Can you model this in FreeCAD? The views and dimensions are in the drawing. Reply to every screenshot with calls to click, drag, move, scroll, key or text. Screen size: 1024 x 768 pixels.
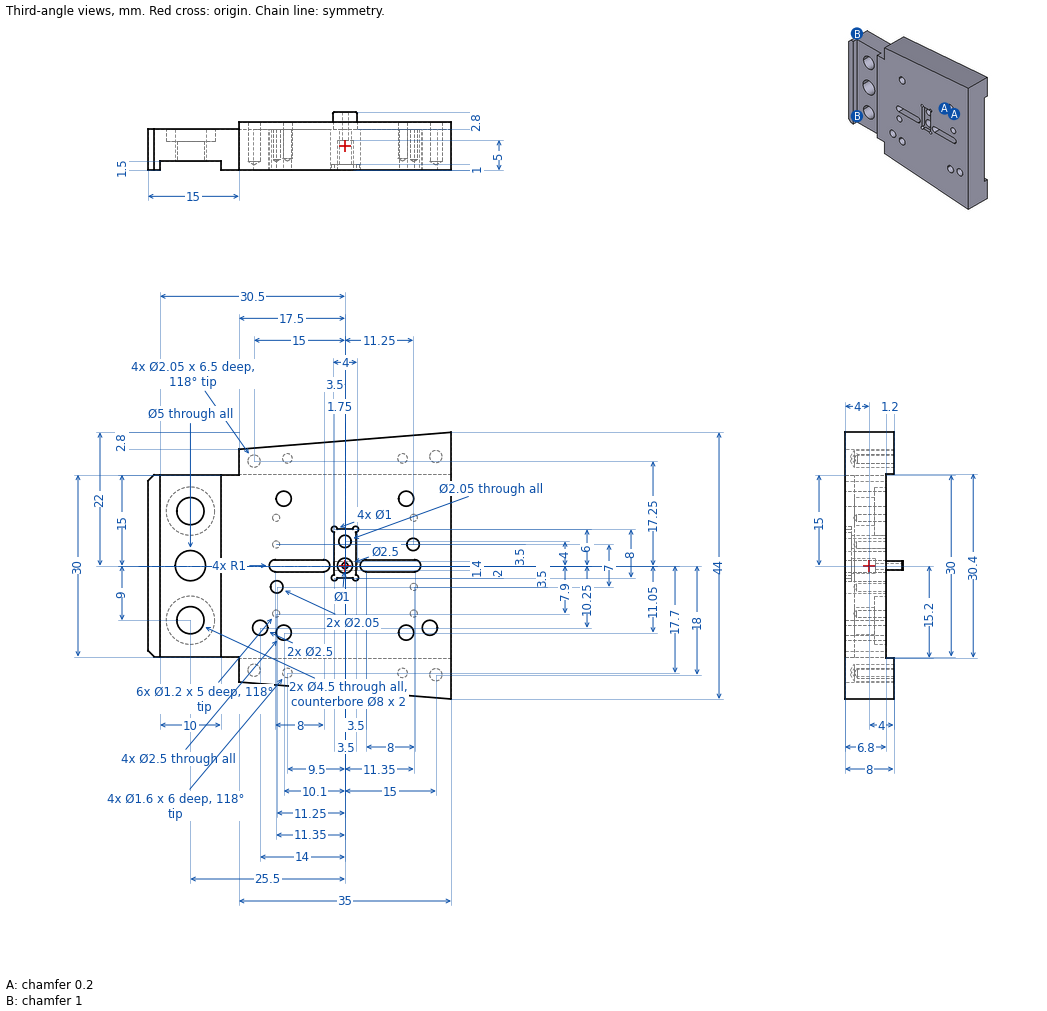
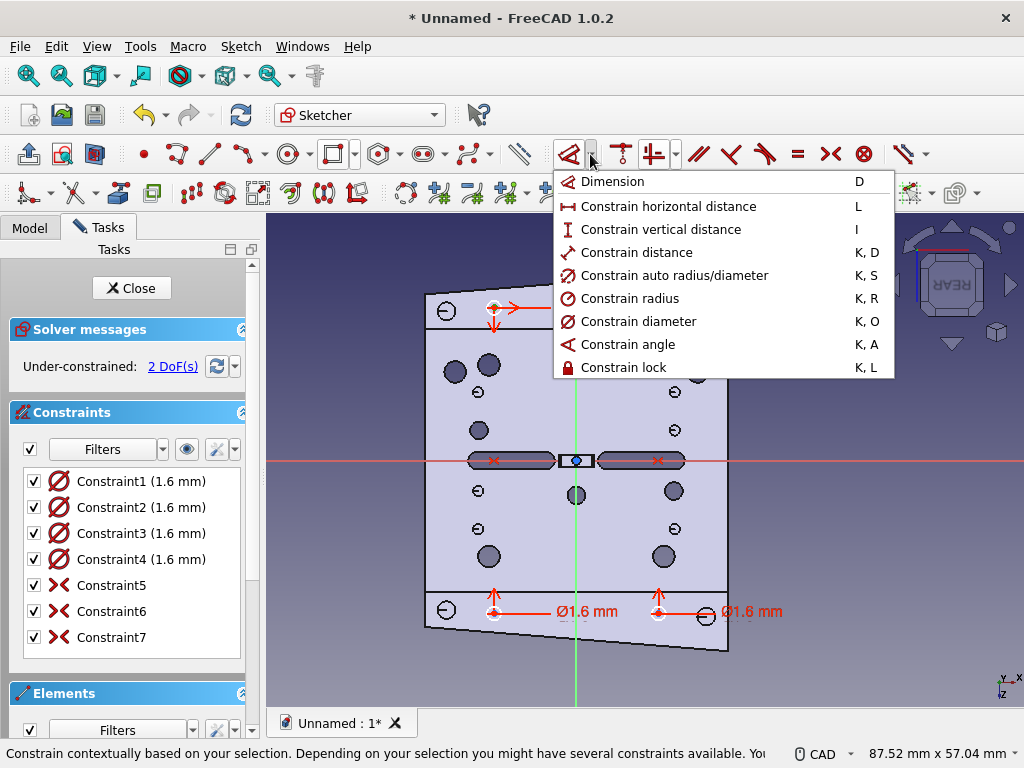
click(724, 206)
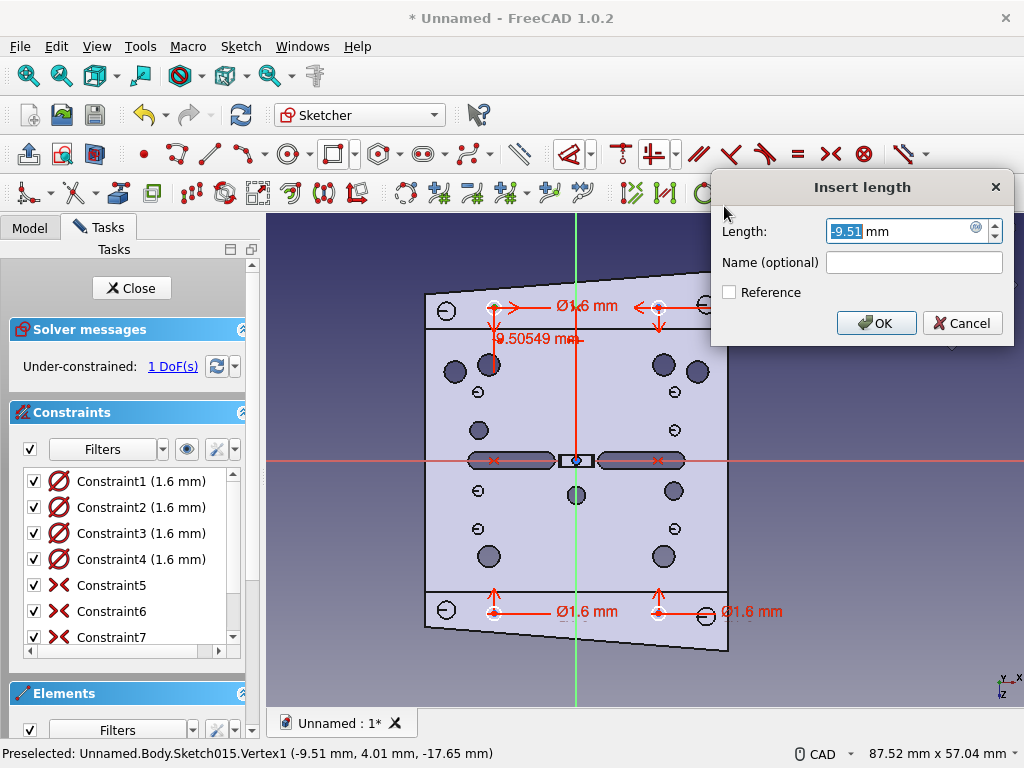
text(-9.5)
key(Return)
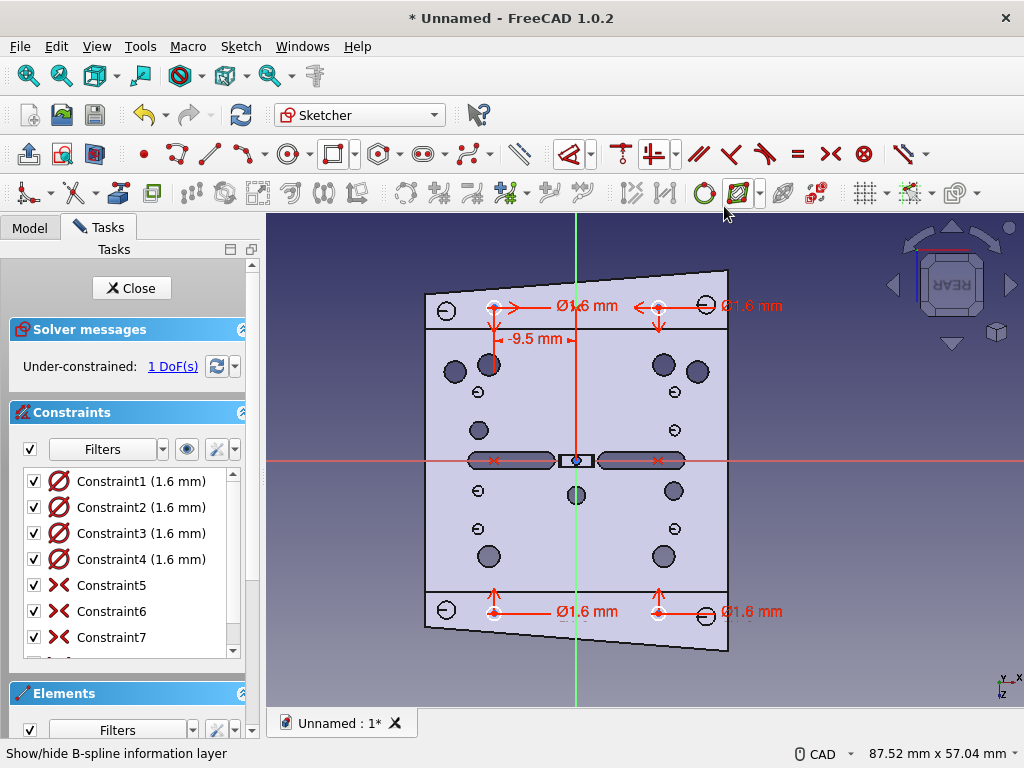
click(494, 308)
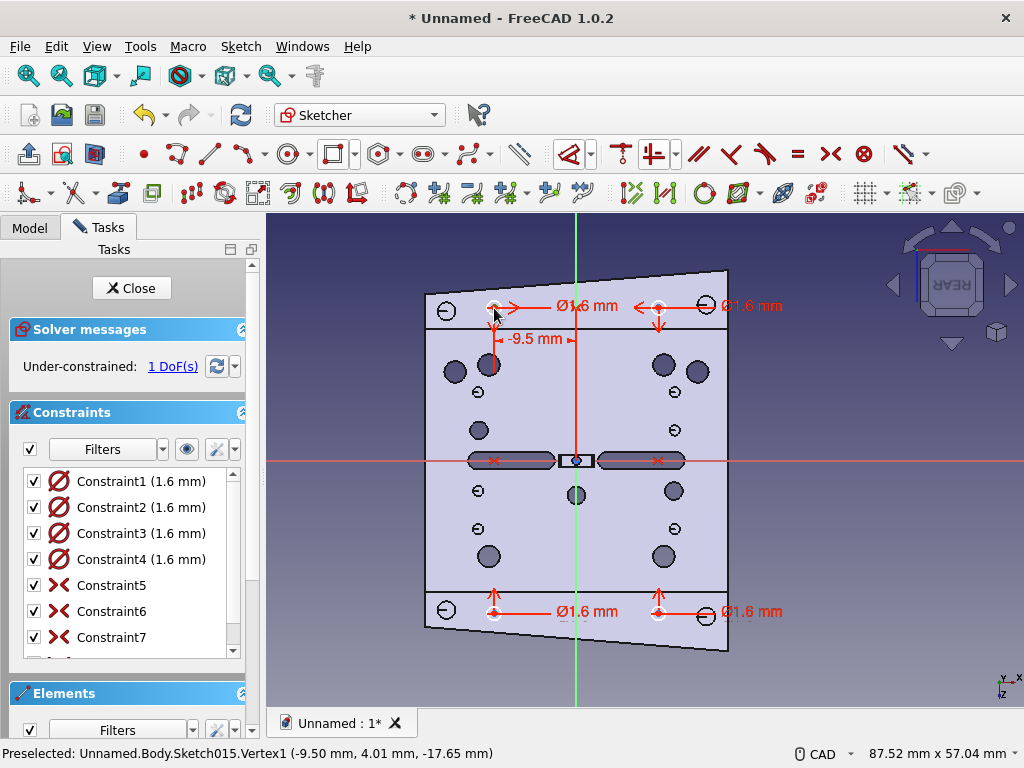
click(590, 154)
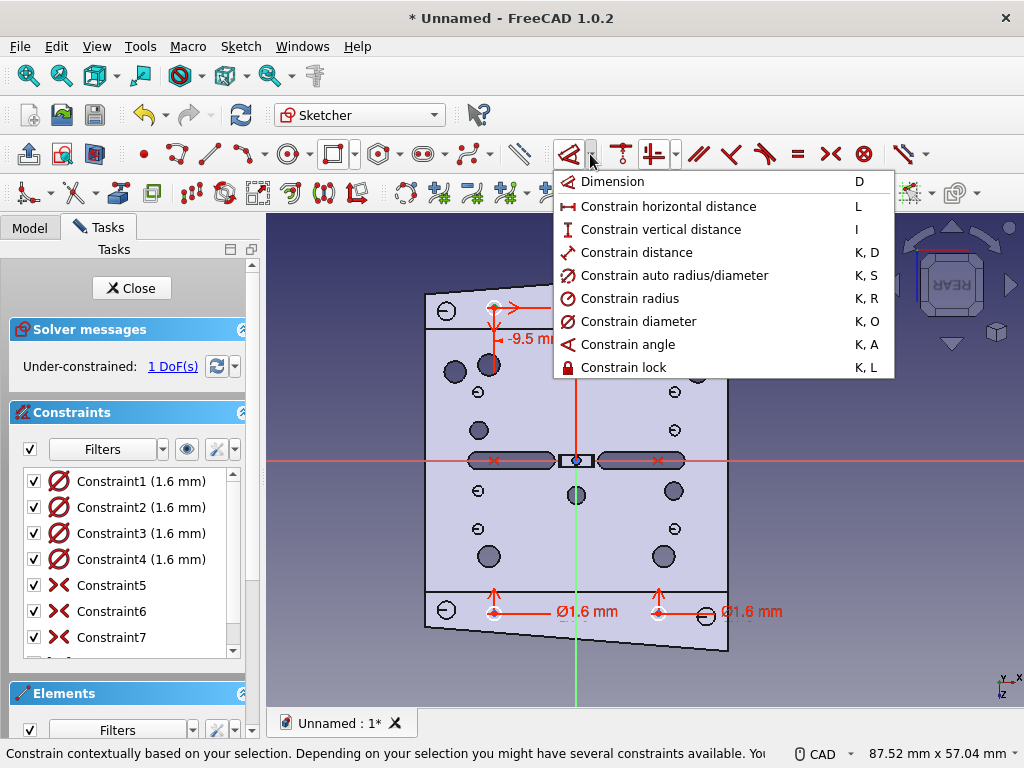
click(724, 230)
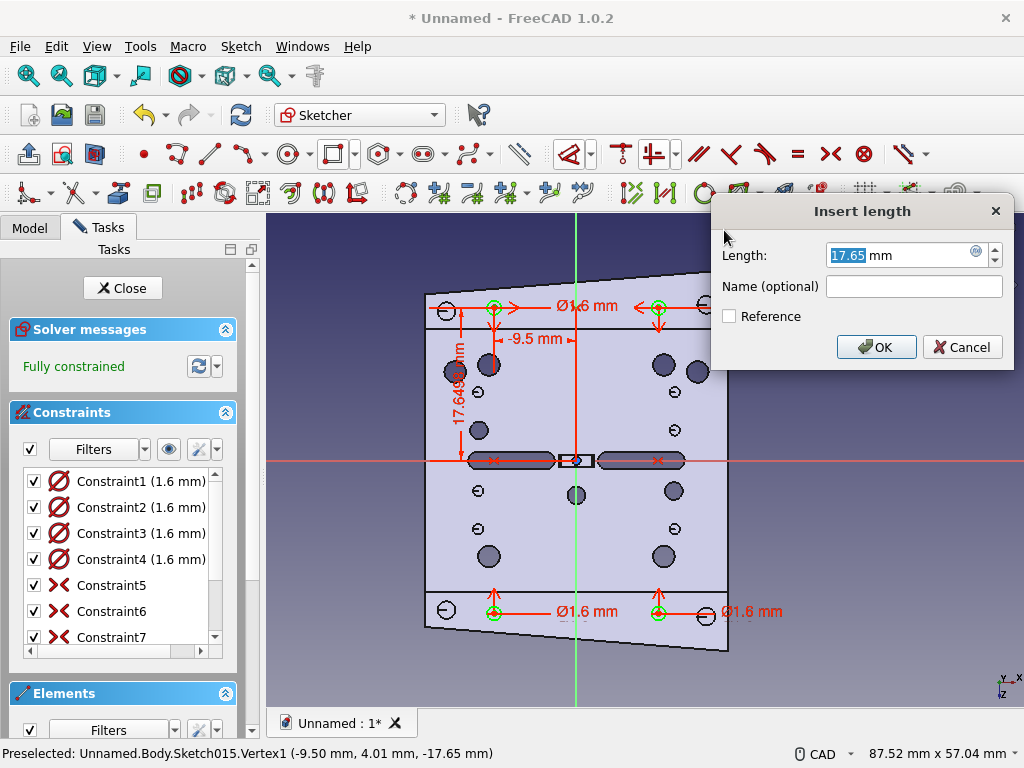
text(17.7)
key(Return)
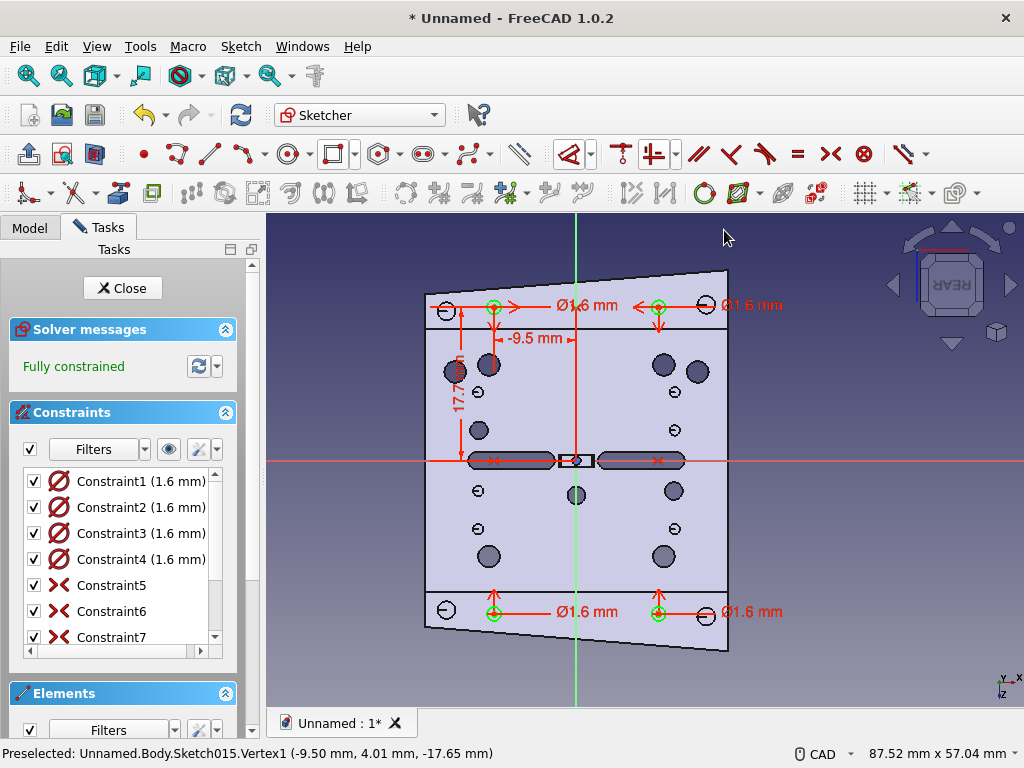
click(123, 288)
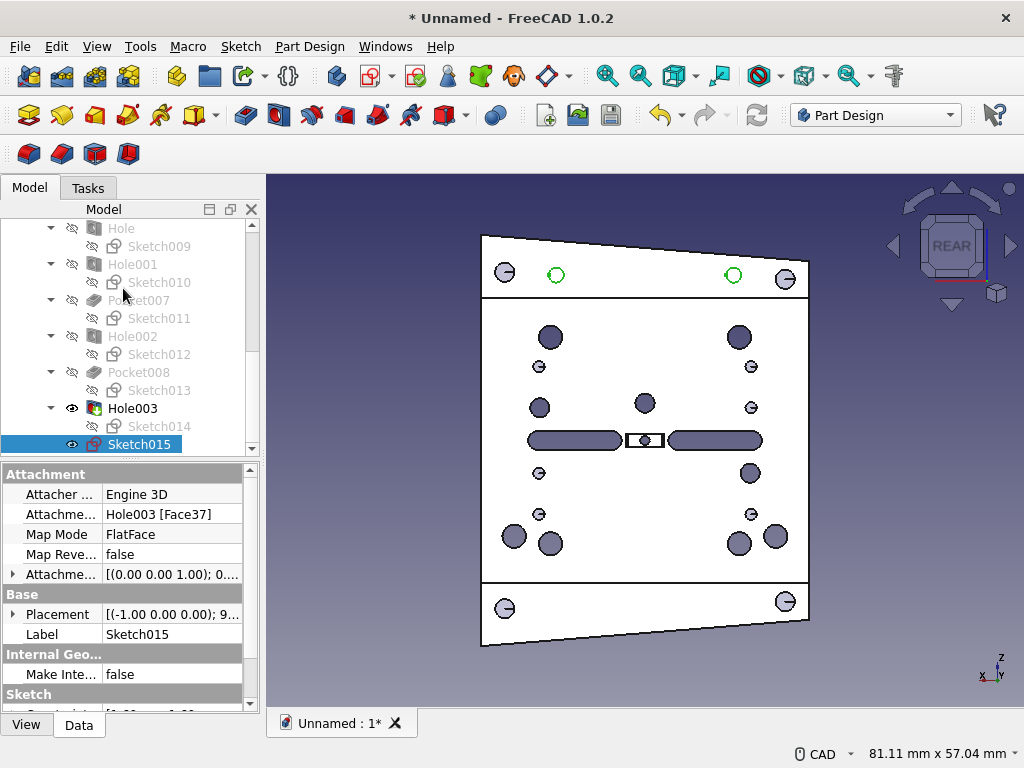
click(279, 116)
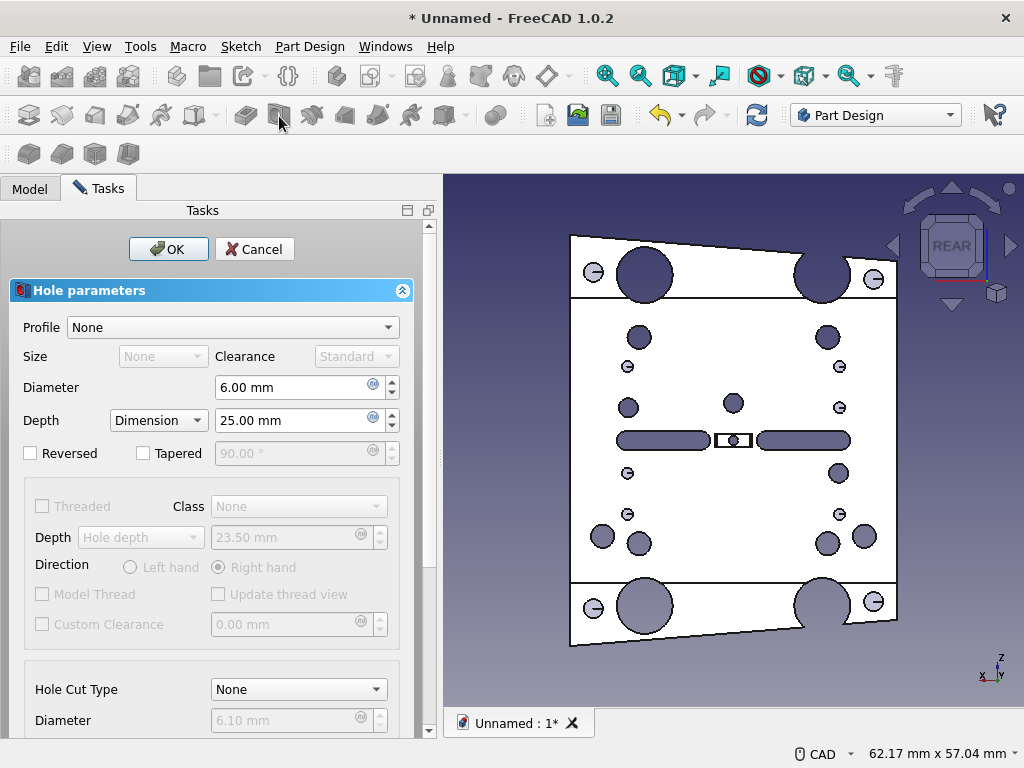
triple_click(300, 388)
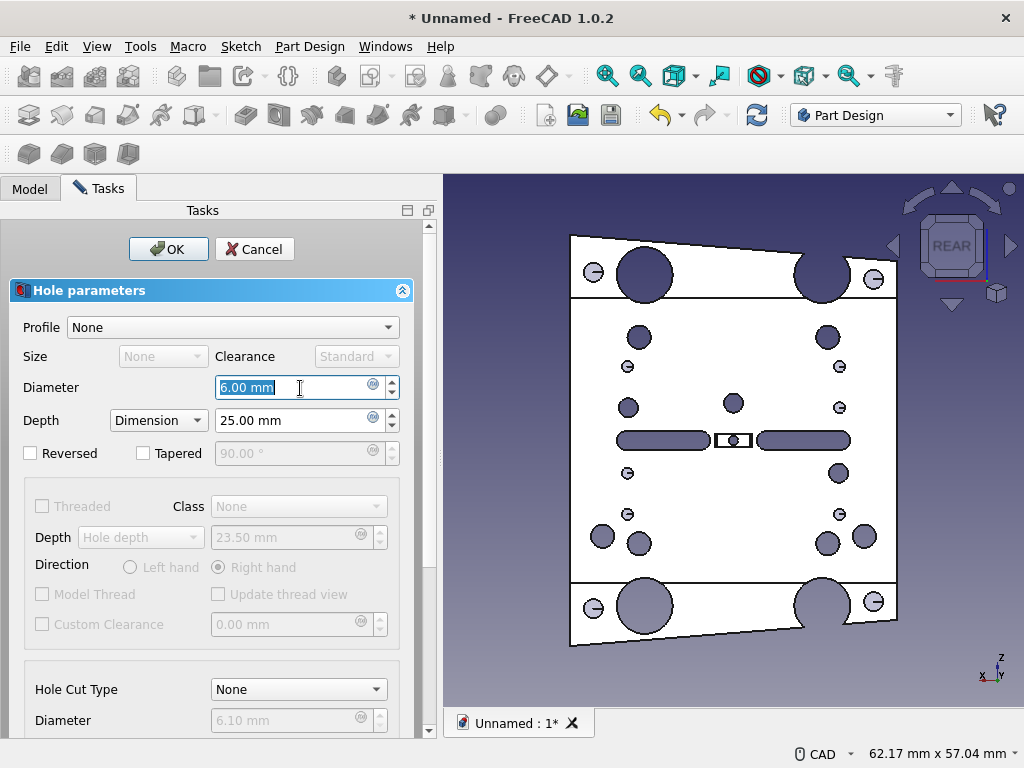
text(1.6)
key(Tab)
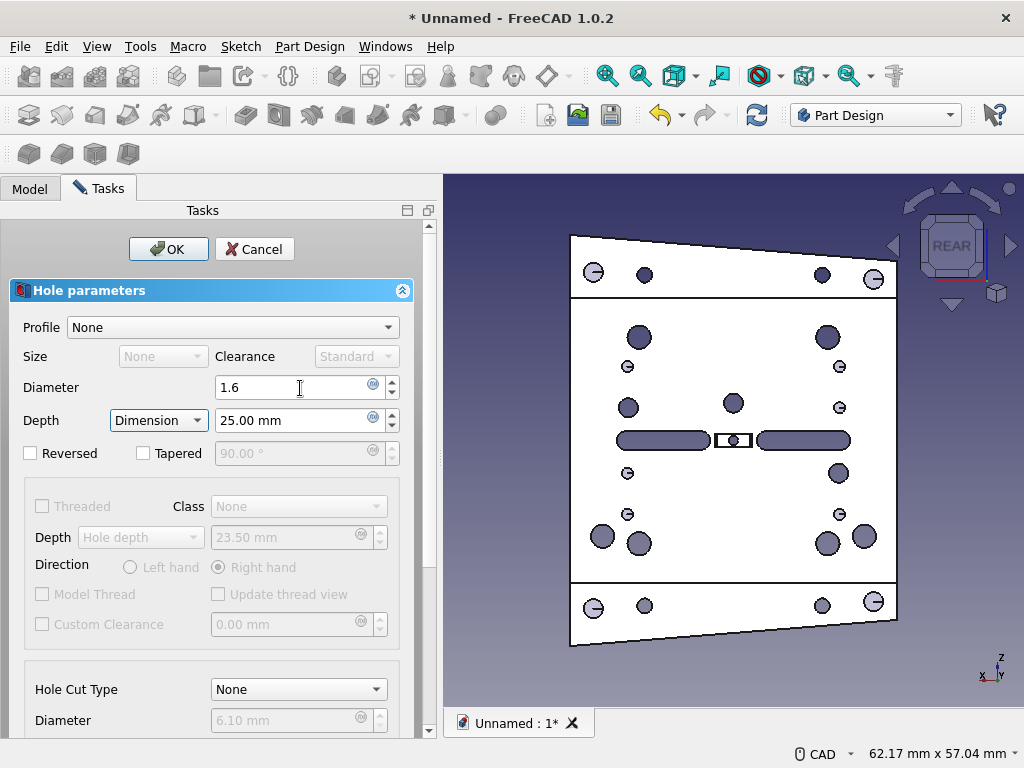
triple_click(300, 420)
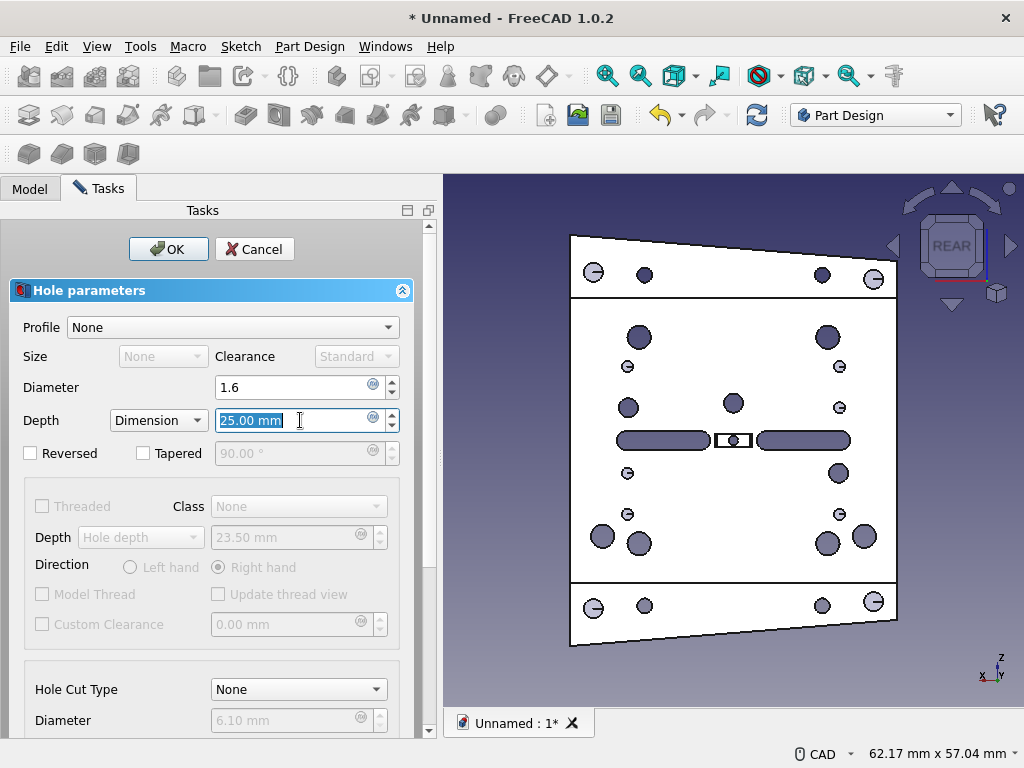
text(6)
key(Tab)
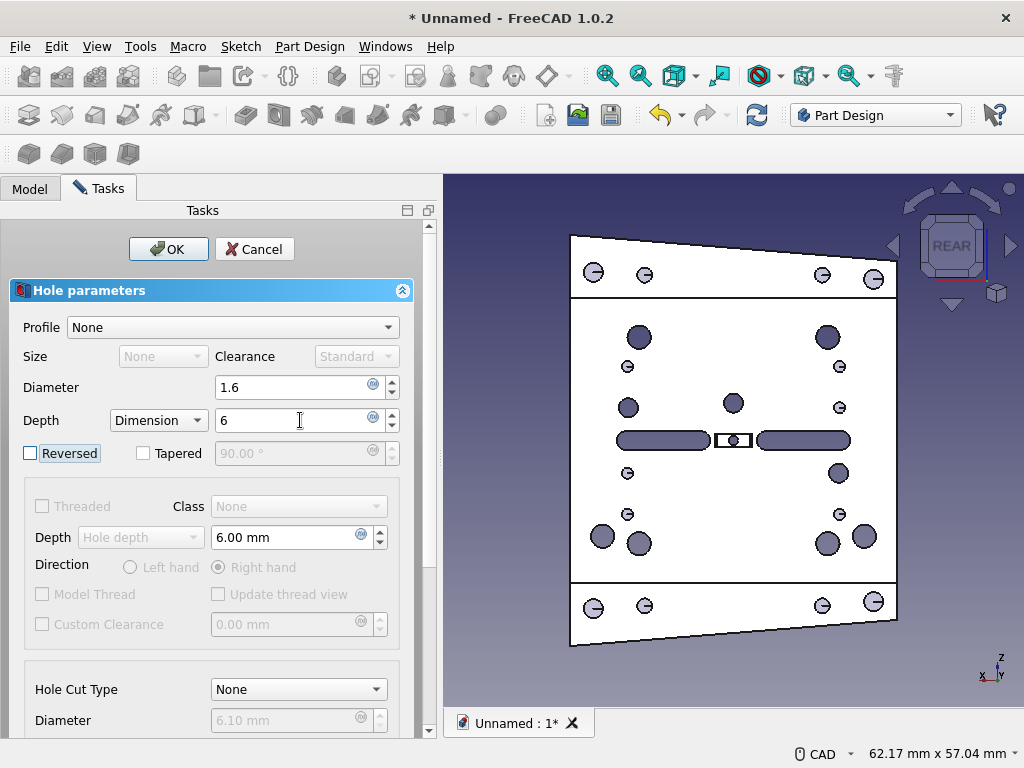
click(169, 249)